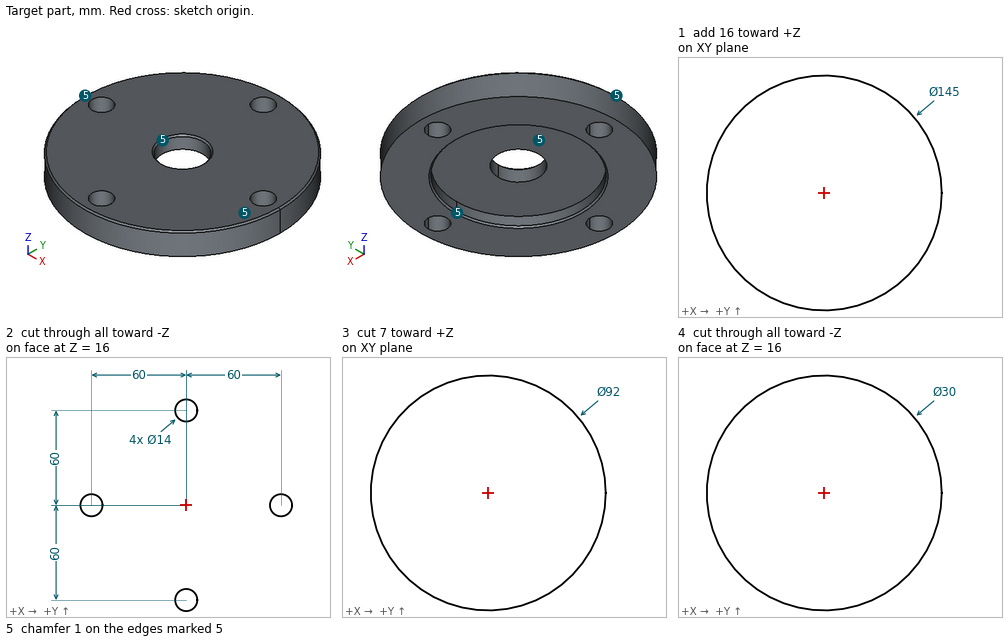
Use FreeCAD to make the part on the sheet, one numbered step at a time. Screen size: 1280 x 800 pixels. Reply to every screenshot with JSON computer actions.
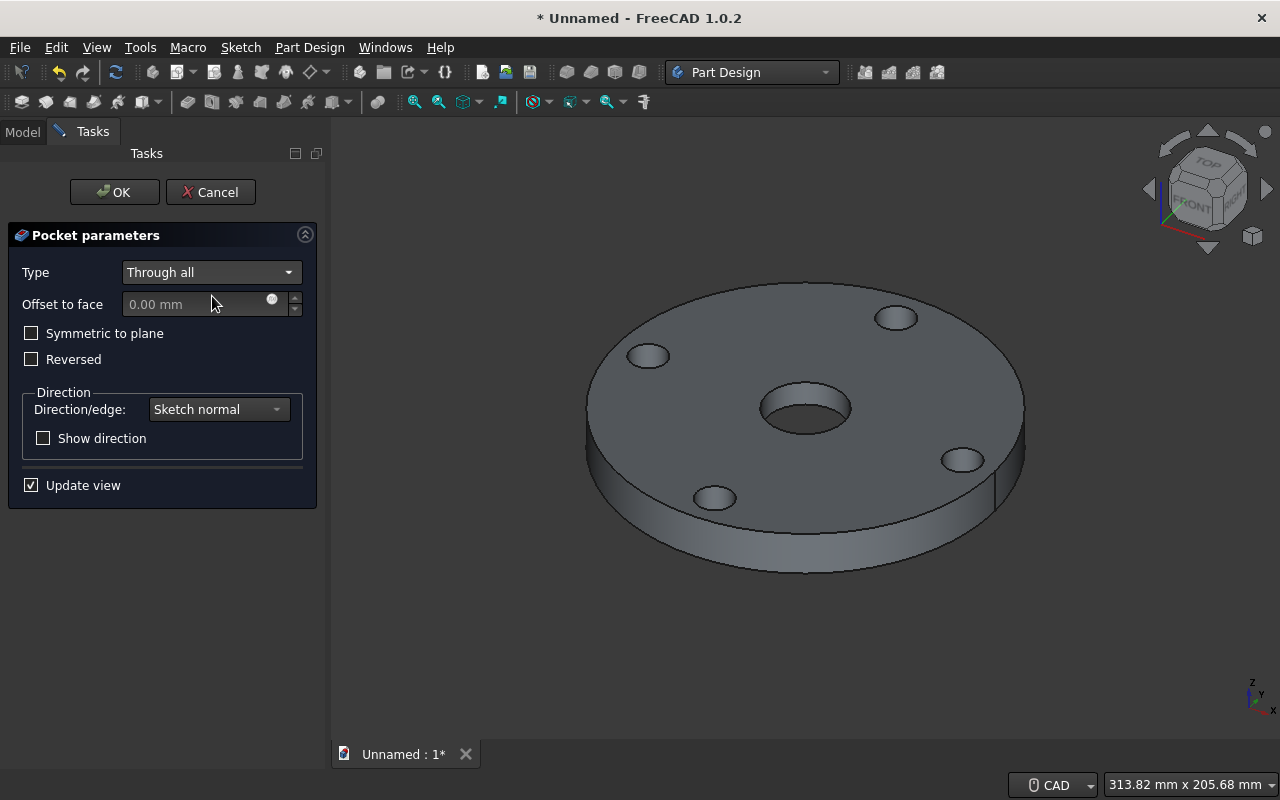
{"action": "left_click", "coordinate": [115, 192]}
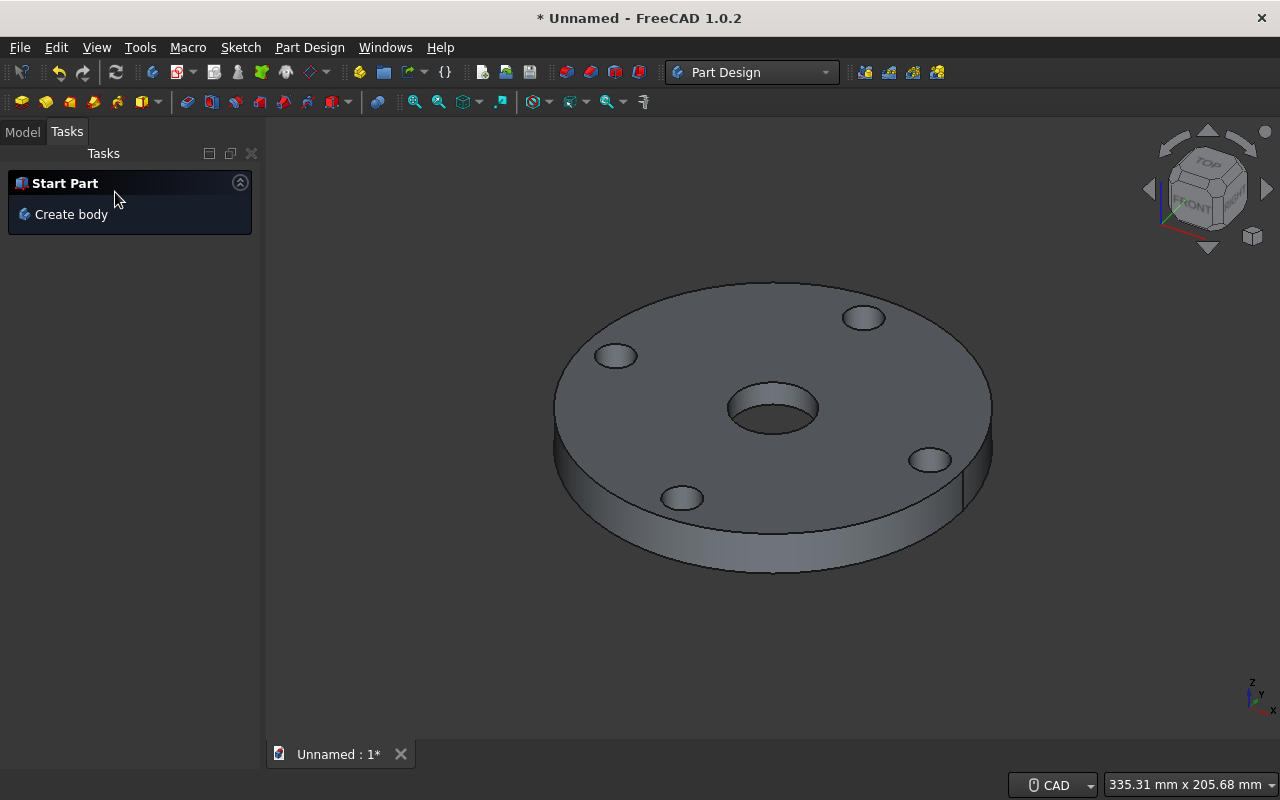
{"action": "left_click", "coordinate": [734, 394]}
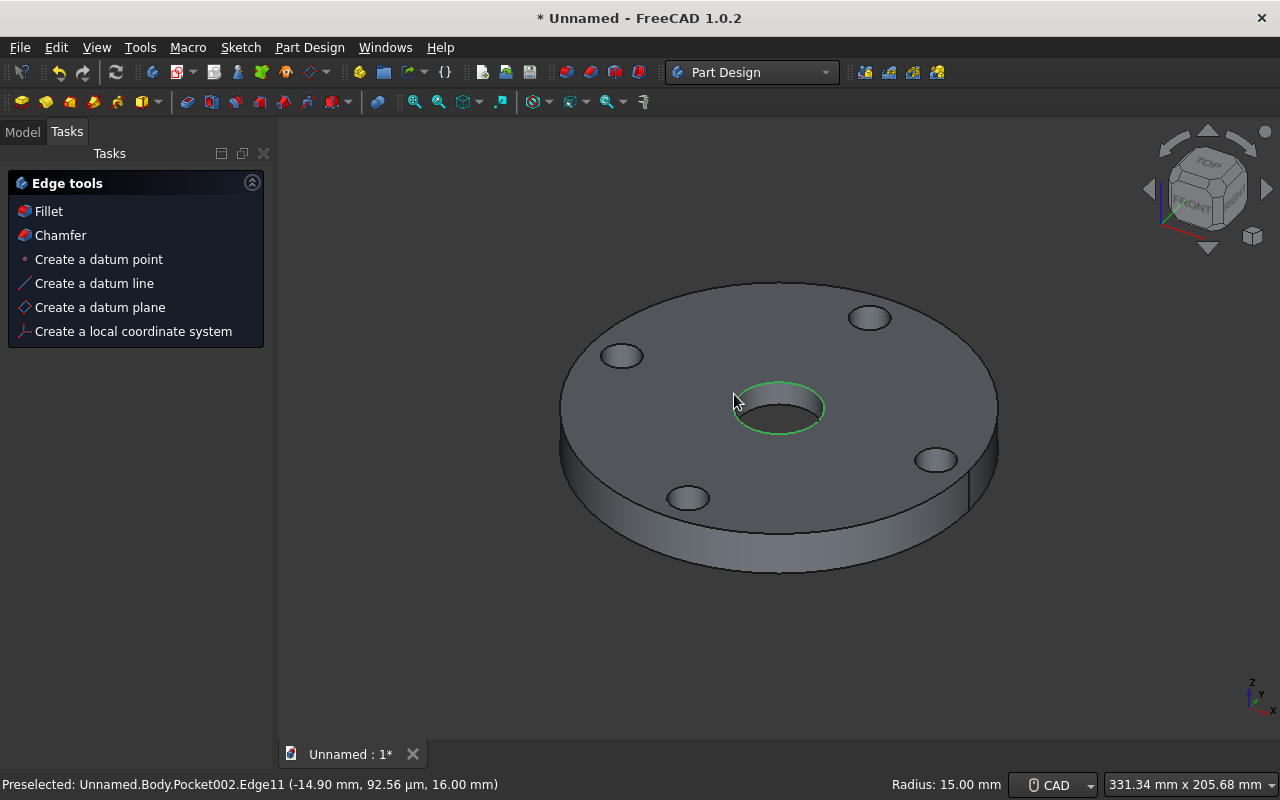
{"action": "left_click", "coordinate": [561, 420], "text": "ctrl"}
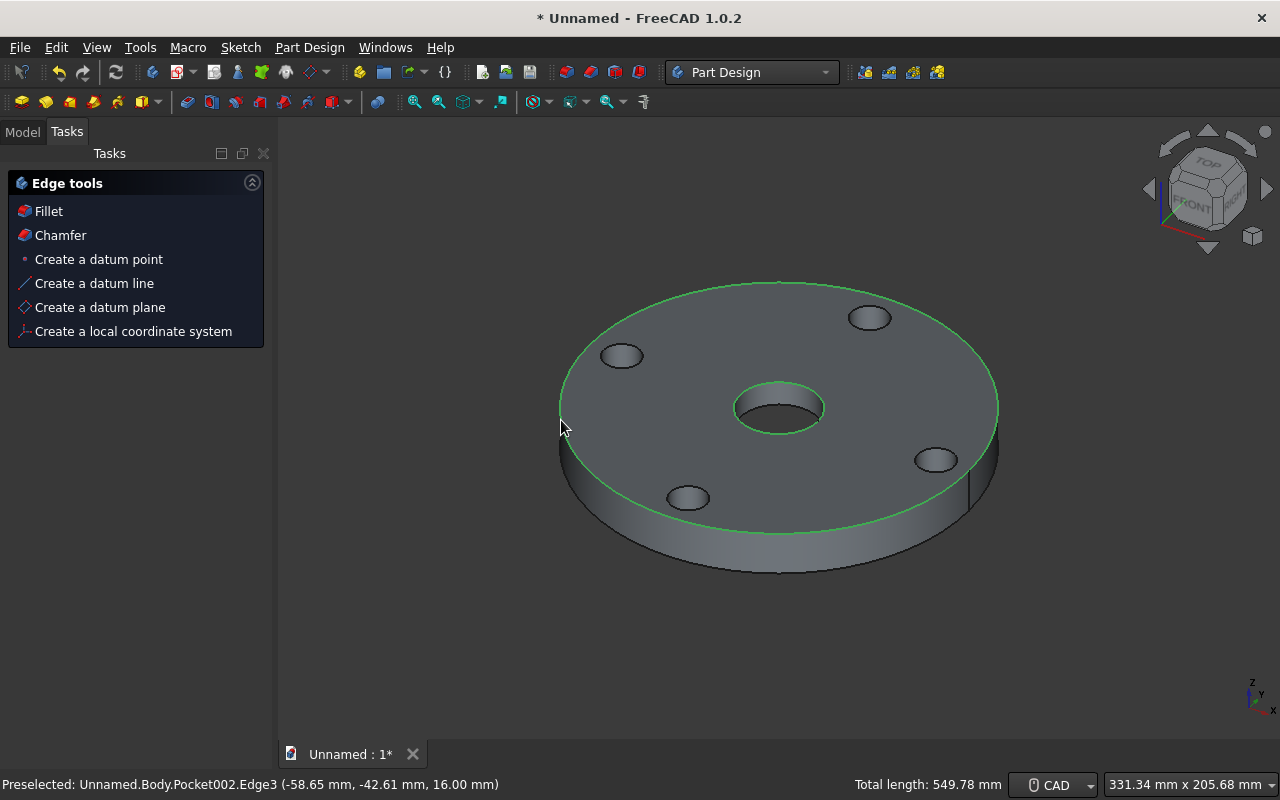
{"action": "key", "text": "0"}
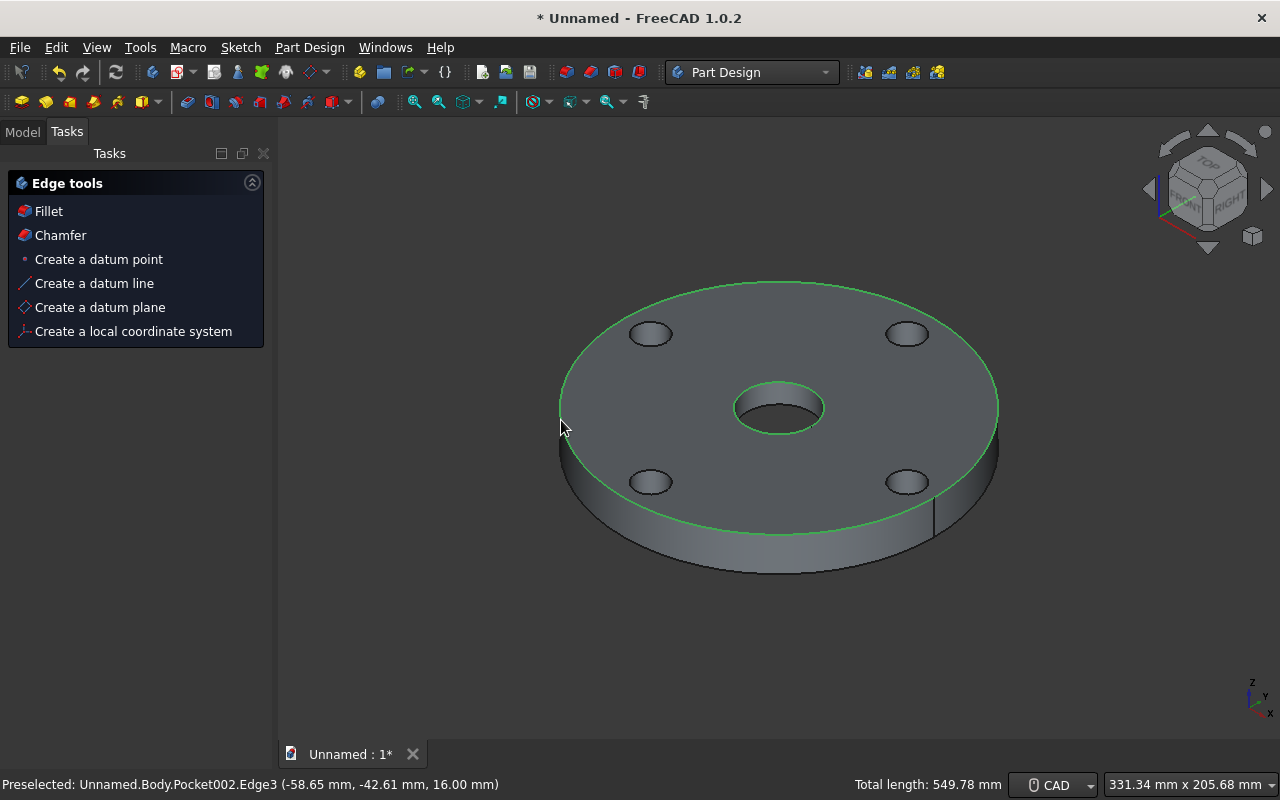
{"action": "key", "text": "2"}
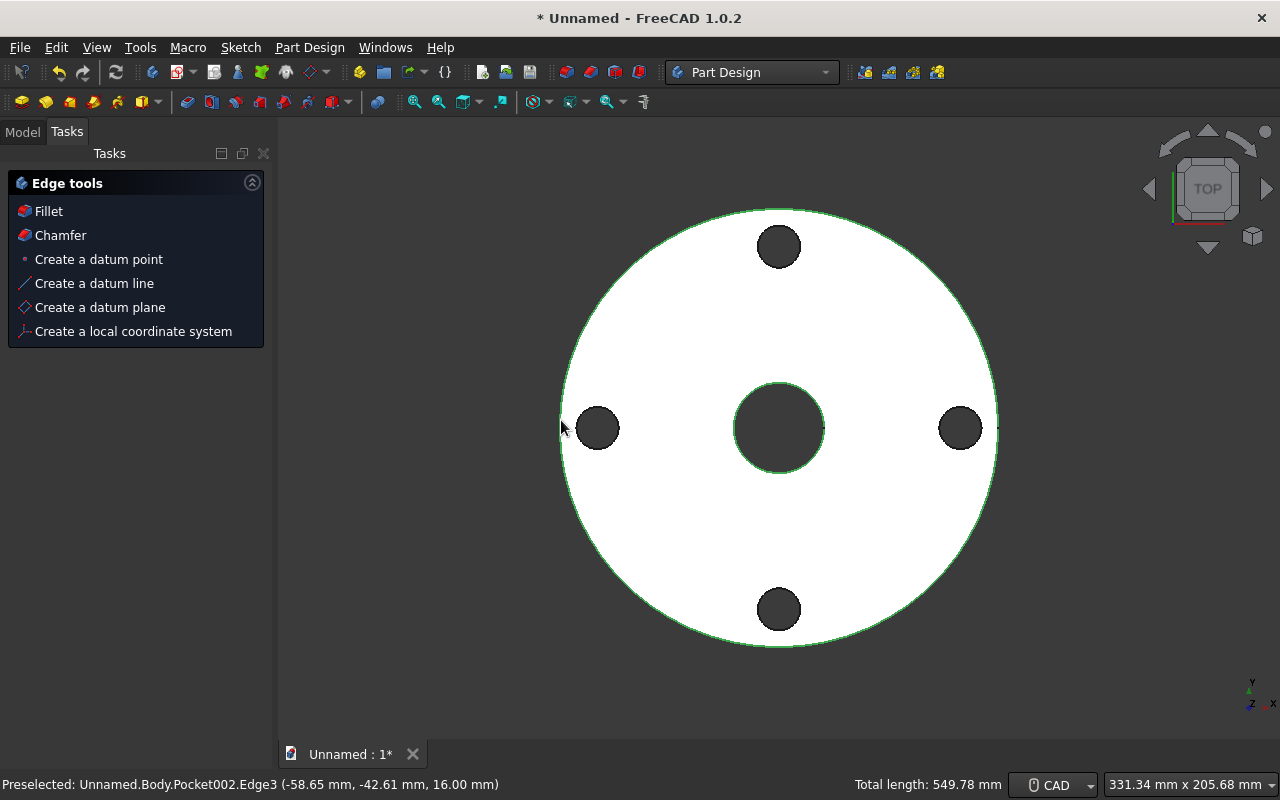
{"action": "key", "text": "1"}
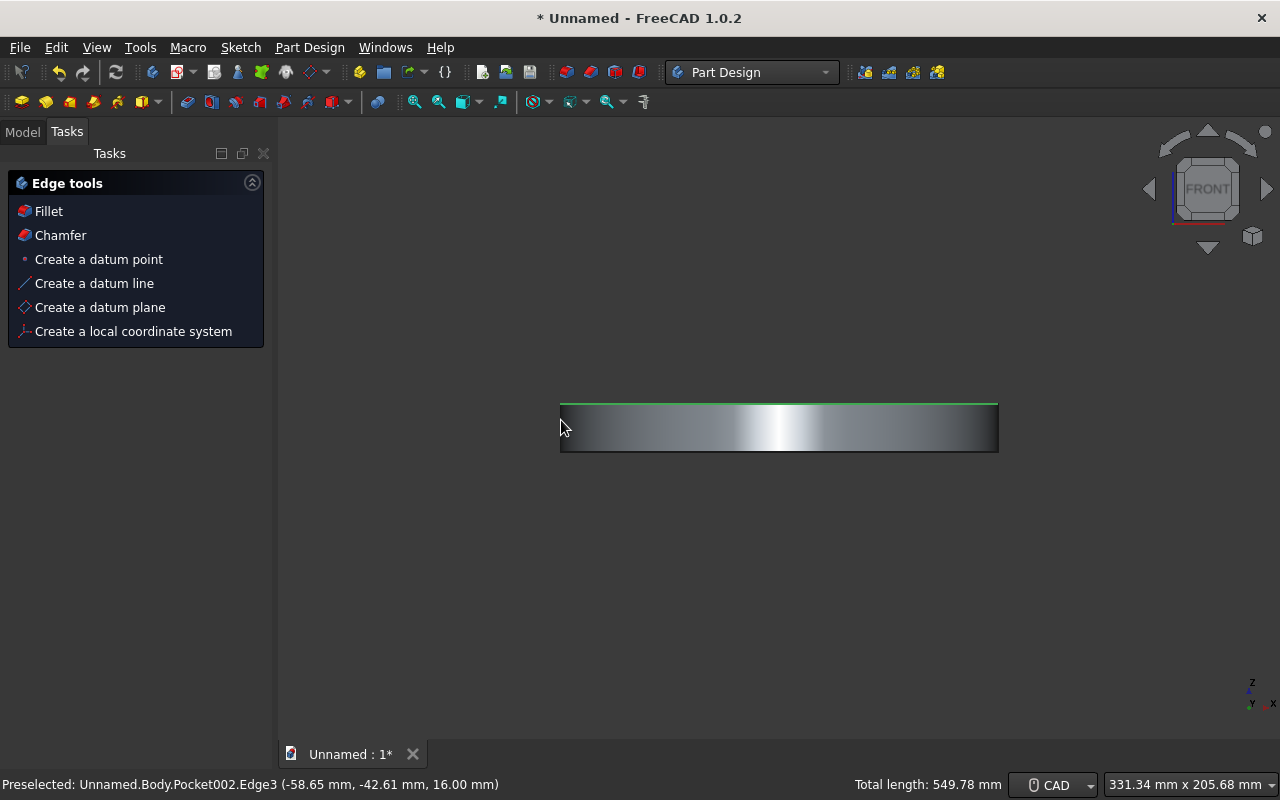
{"action": "key", "text": "v f"}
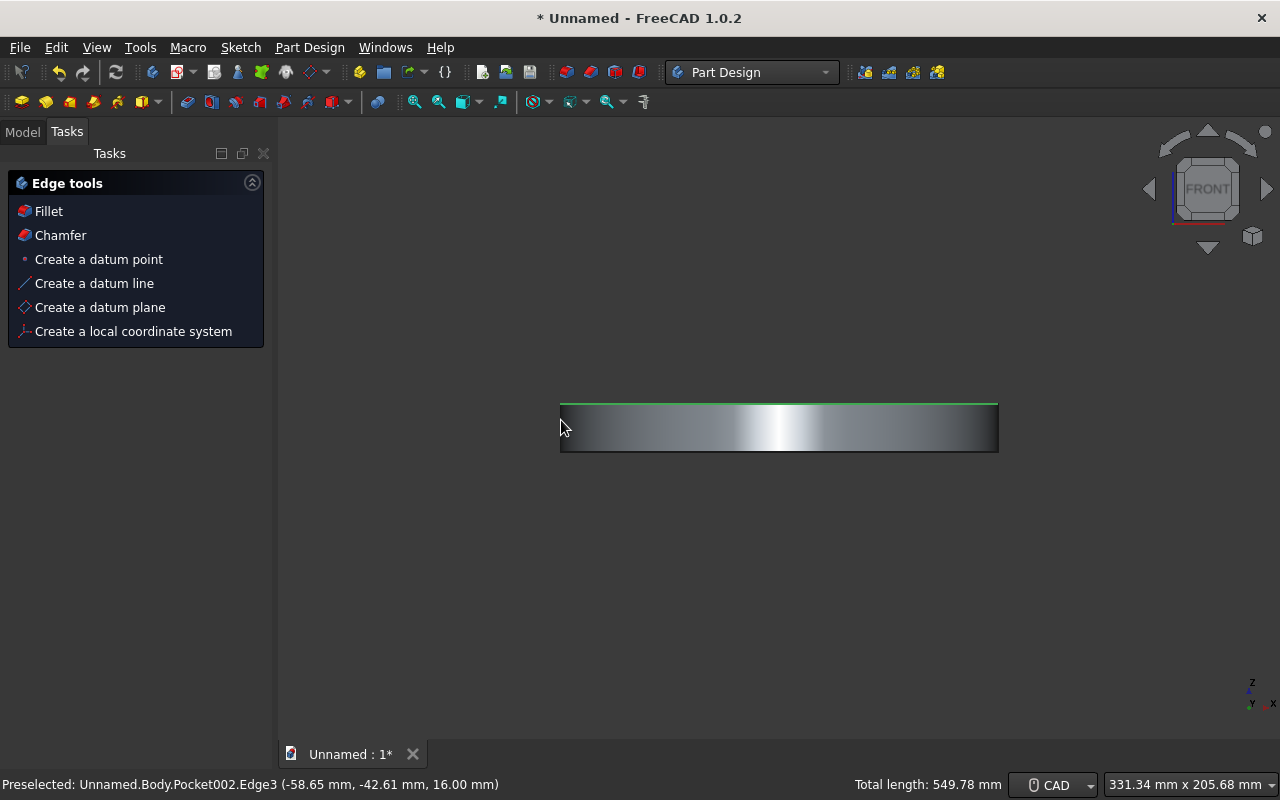
{"action": "key", "text": "3"}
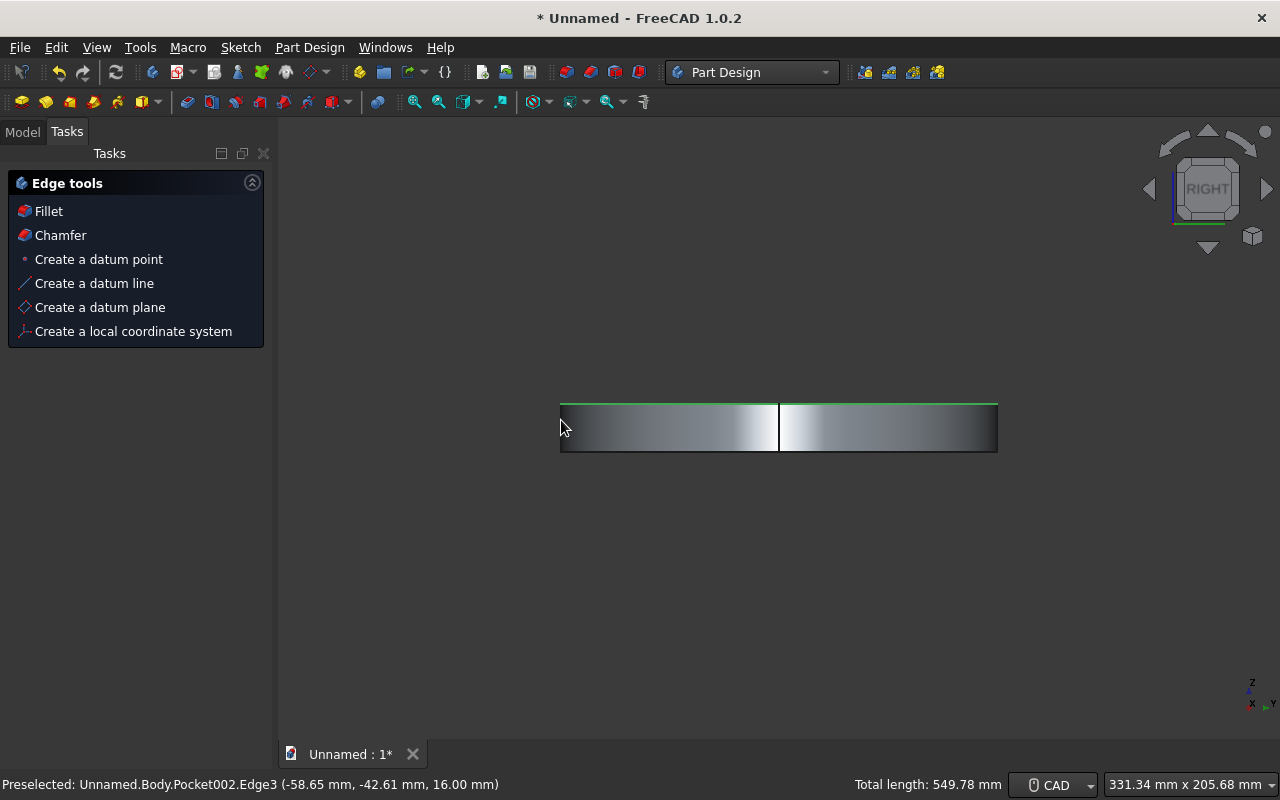
{"action": "key", "text": "v f"}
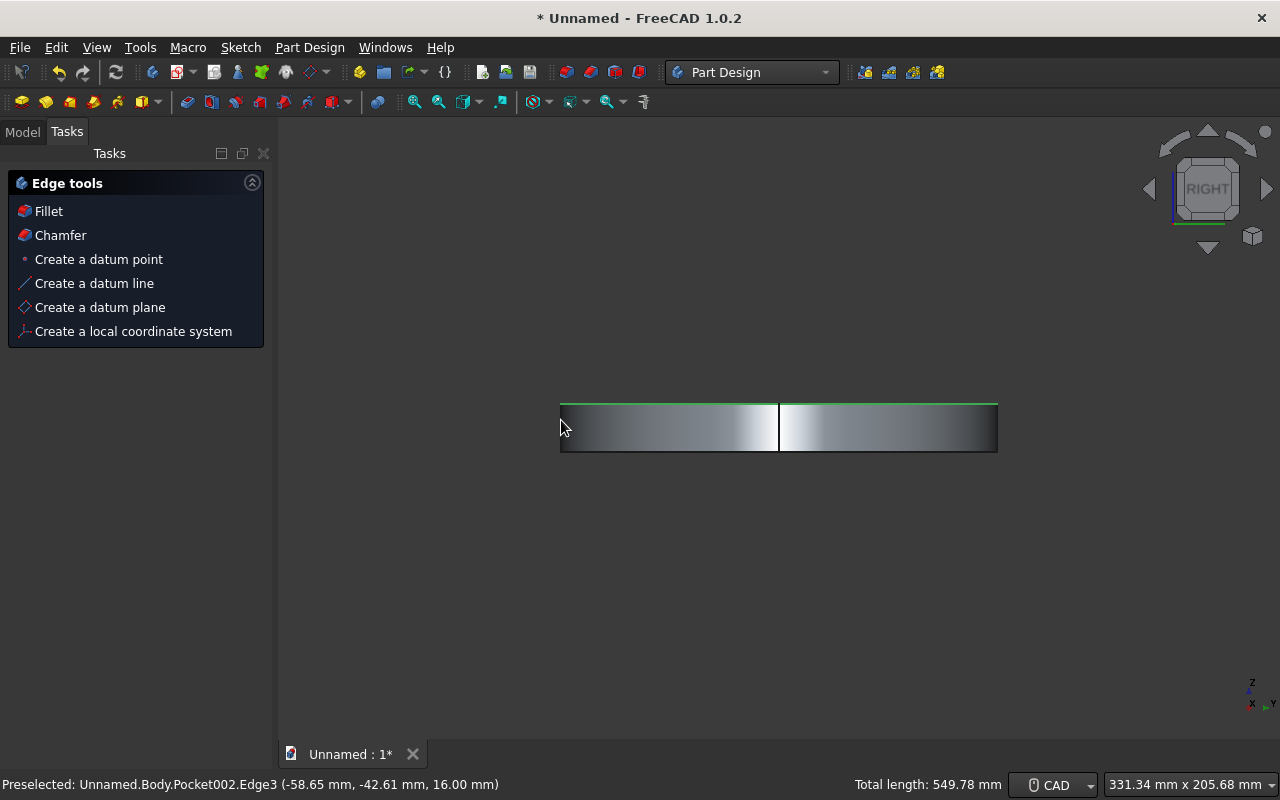
{"action": "key", "text": "5"}